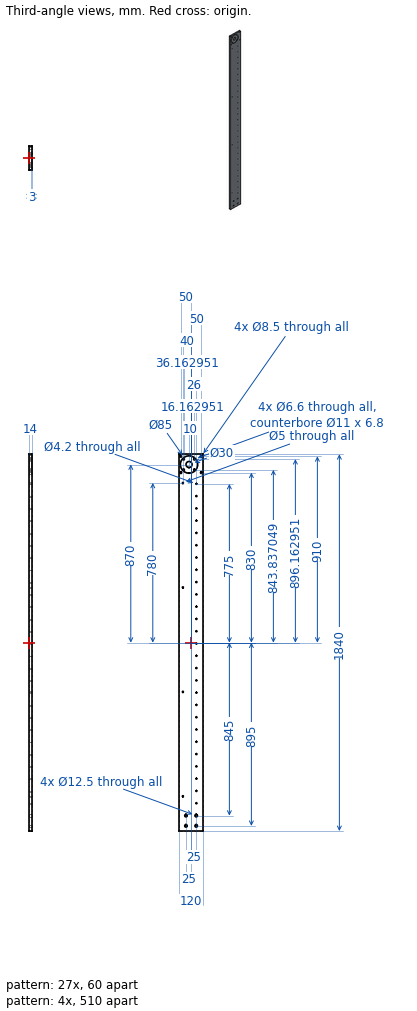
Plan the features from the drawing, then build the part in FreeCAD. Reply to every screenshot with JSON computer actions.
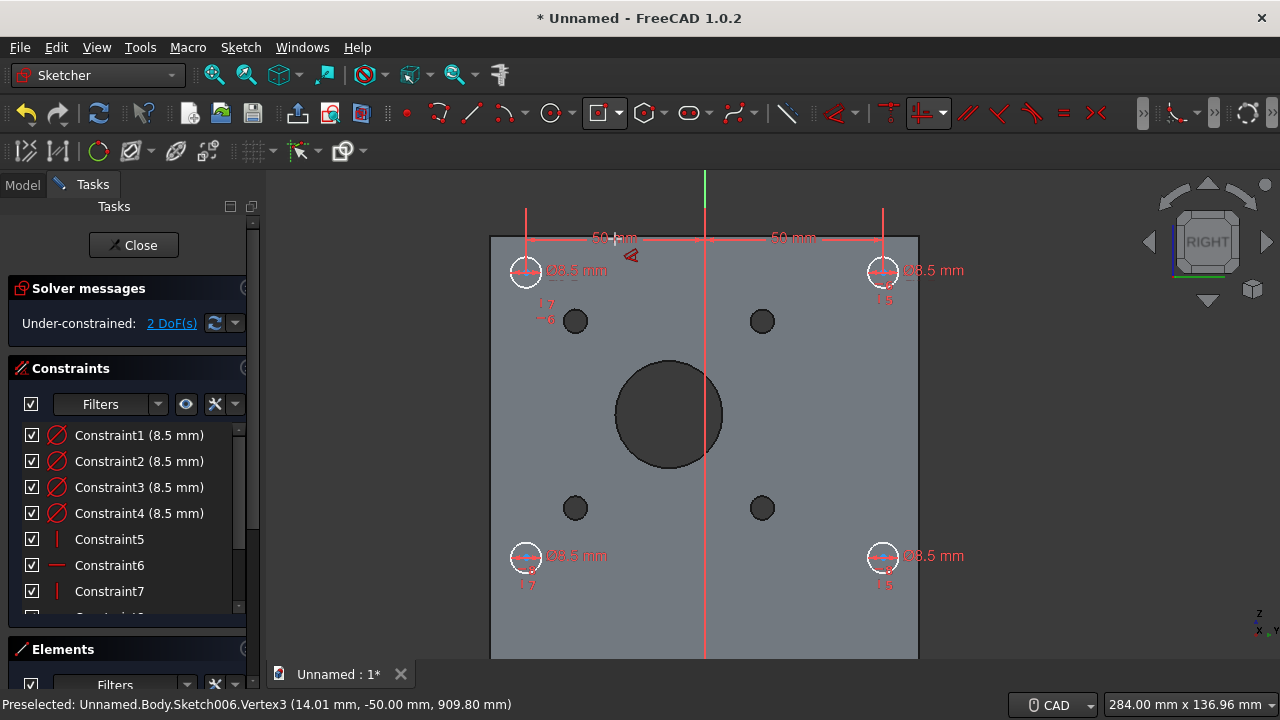
{"action": "left_click", "coordinate": [883, 273]}
{"action": "left_click", "coordinate": [917, 452]}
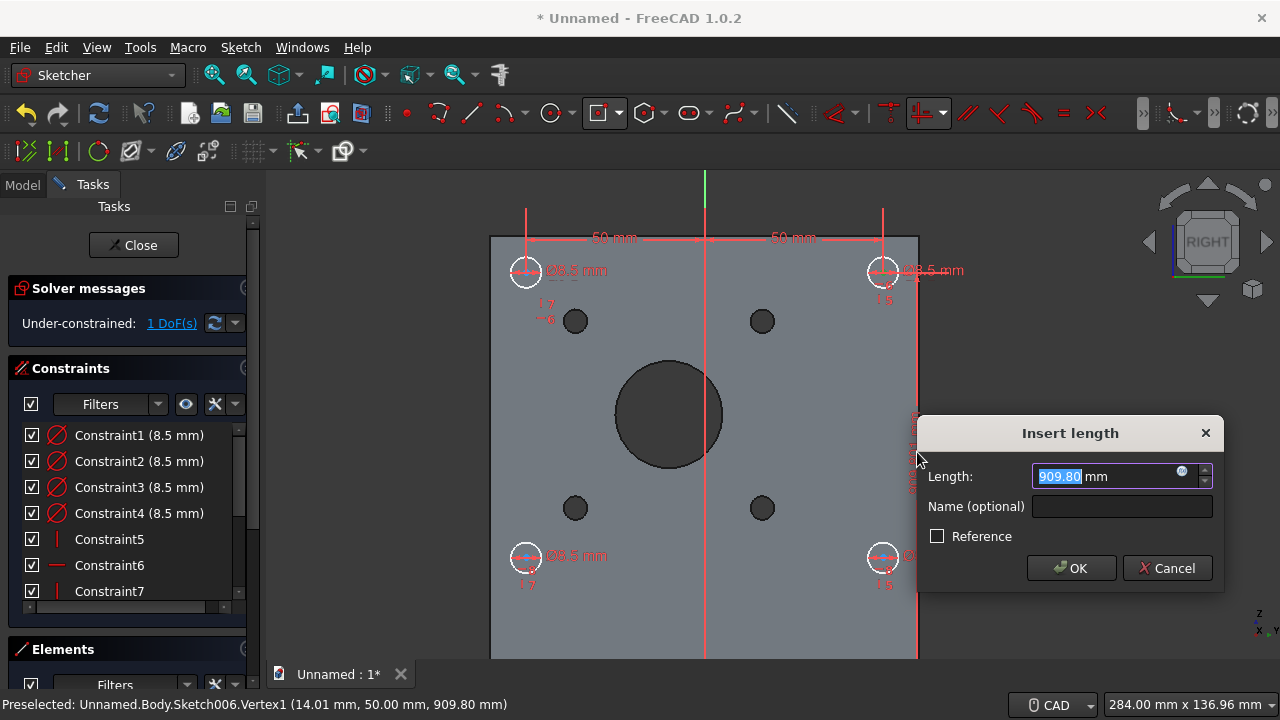
{"action": "type", "text": "910"}
{"action": "key", "text": "Return"}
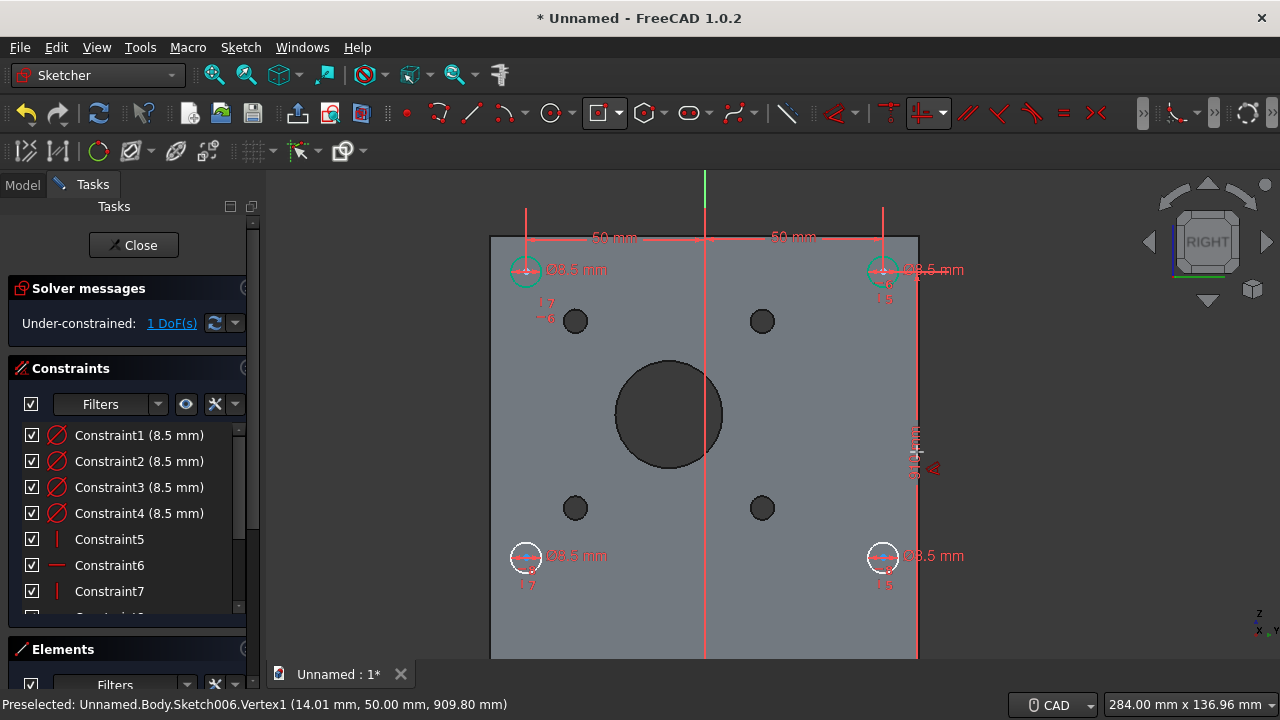
{"action": "left_click", "coordinate": [883, 558]}
{"action": "left_click", "coordinate": [917, 594]}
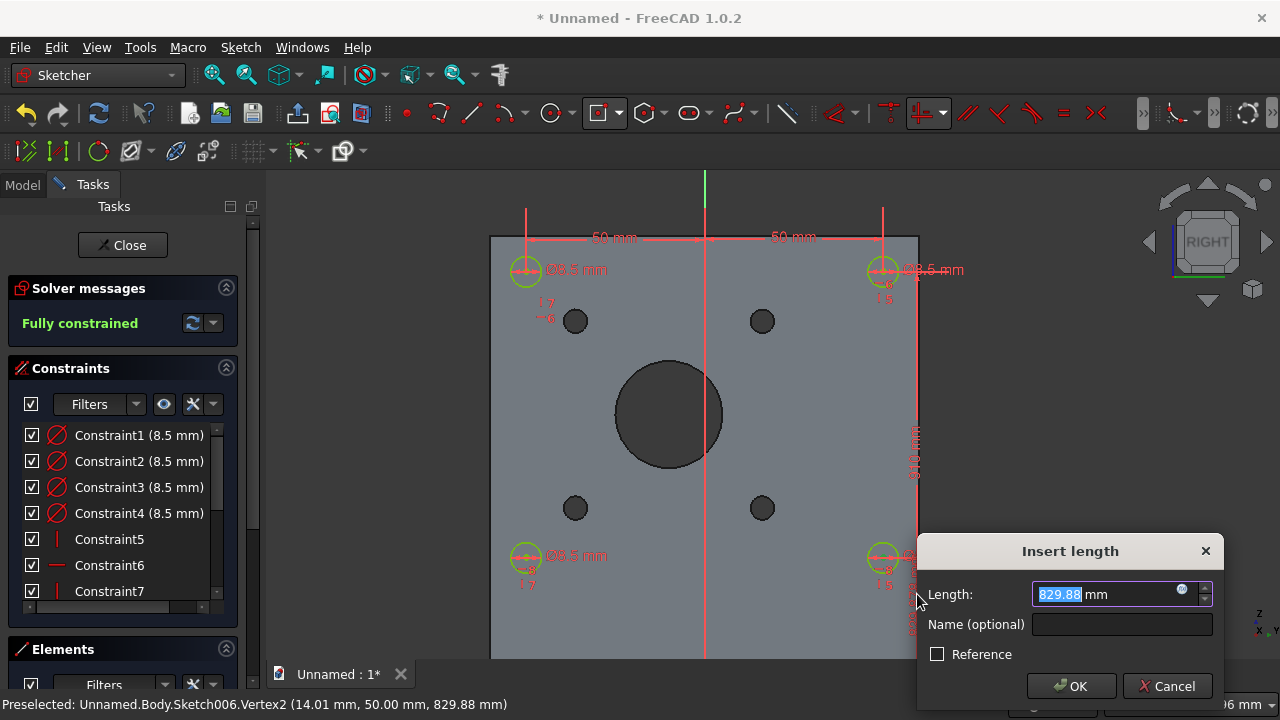
{"action": "type", "text": "830"}
{"action": "key", "text": "Return"}
{"action": "key", "text": "Escape"}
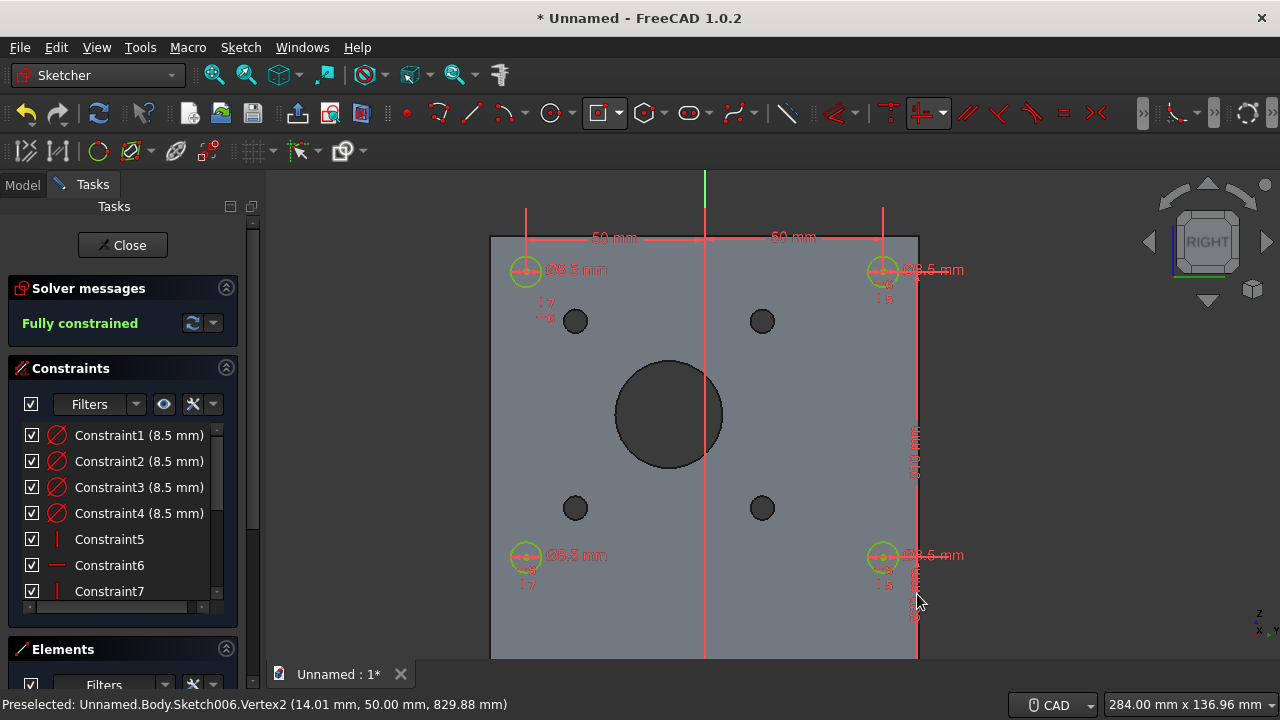
{"action": "left_click", "coordinate": [123, 245]}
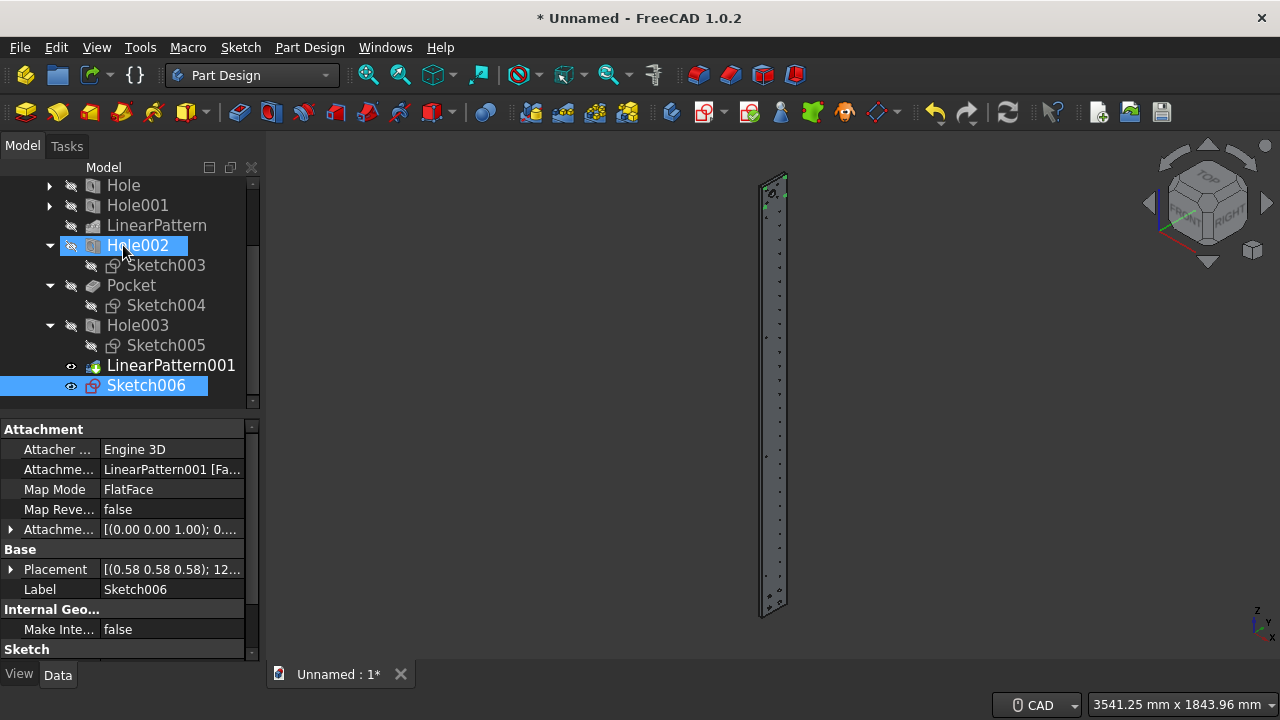
{"action": "left_click", "coordinate": [272, 112]}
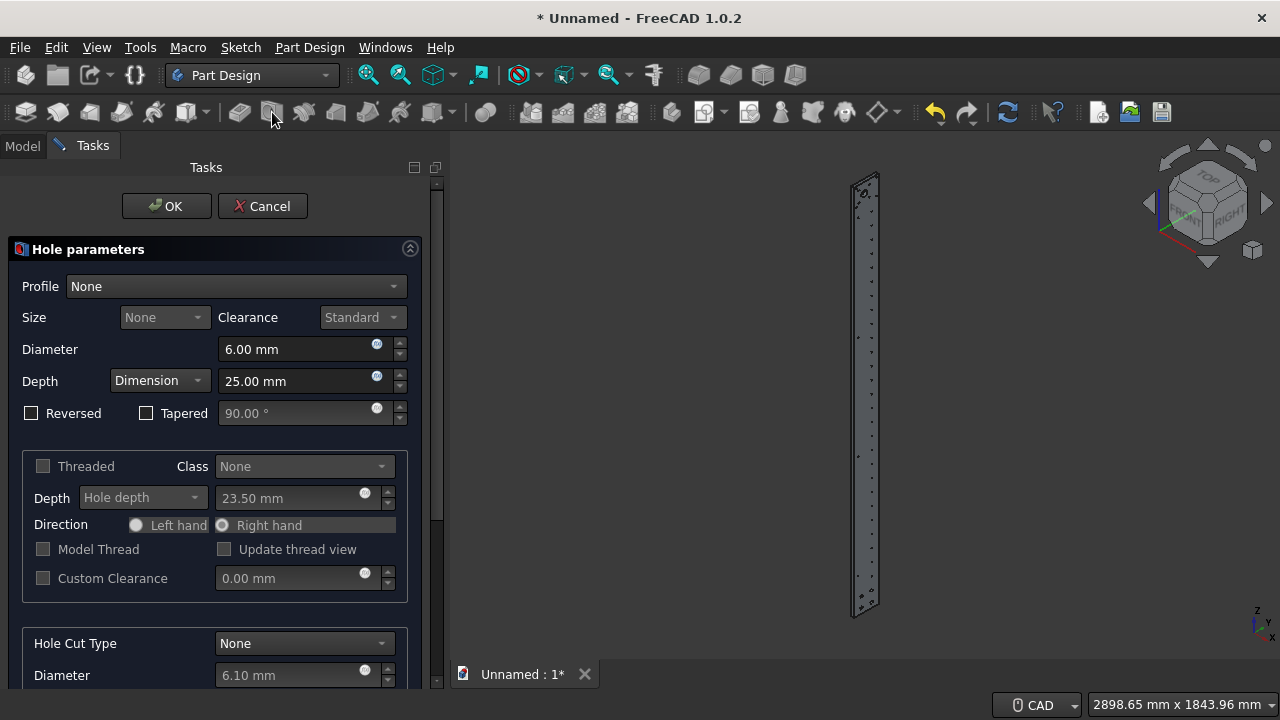
{"action": "triple_click", "coordinate": [305, 349]}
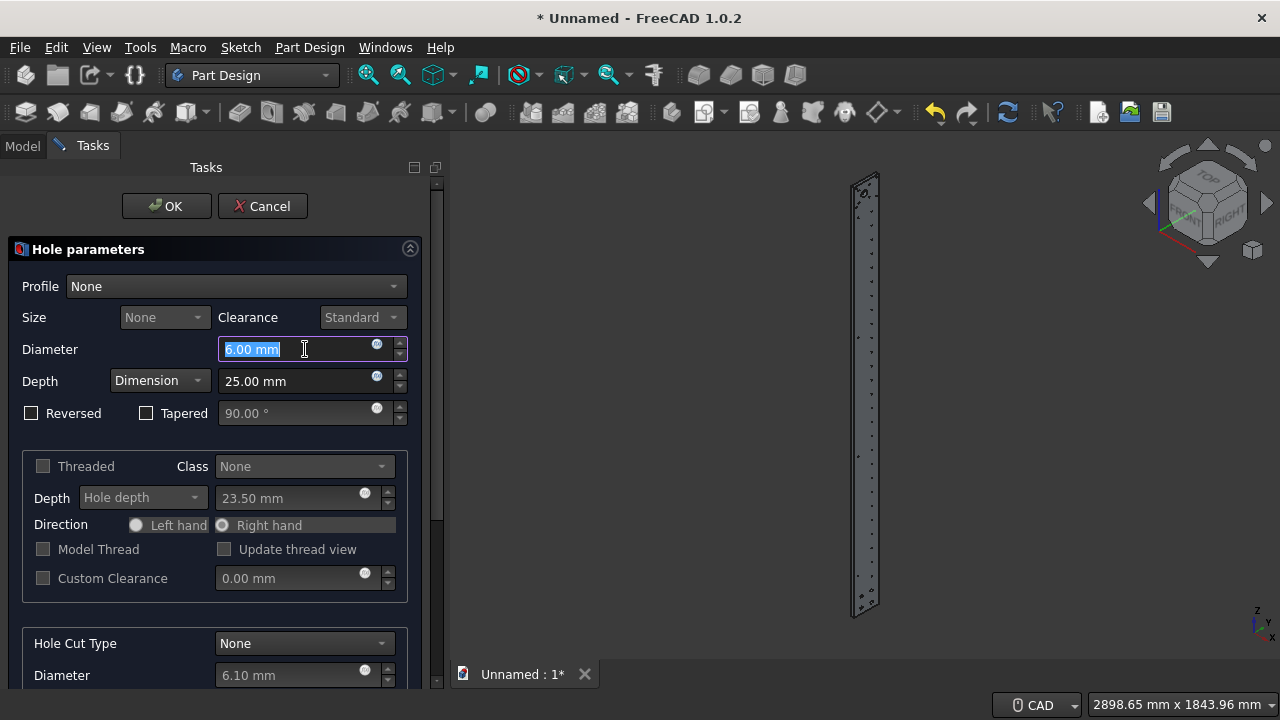
{"action": "type", "text": "8.5"}
{"action": "key", "text": "Tab"}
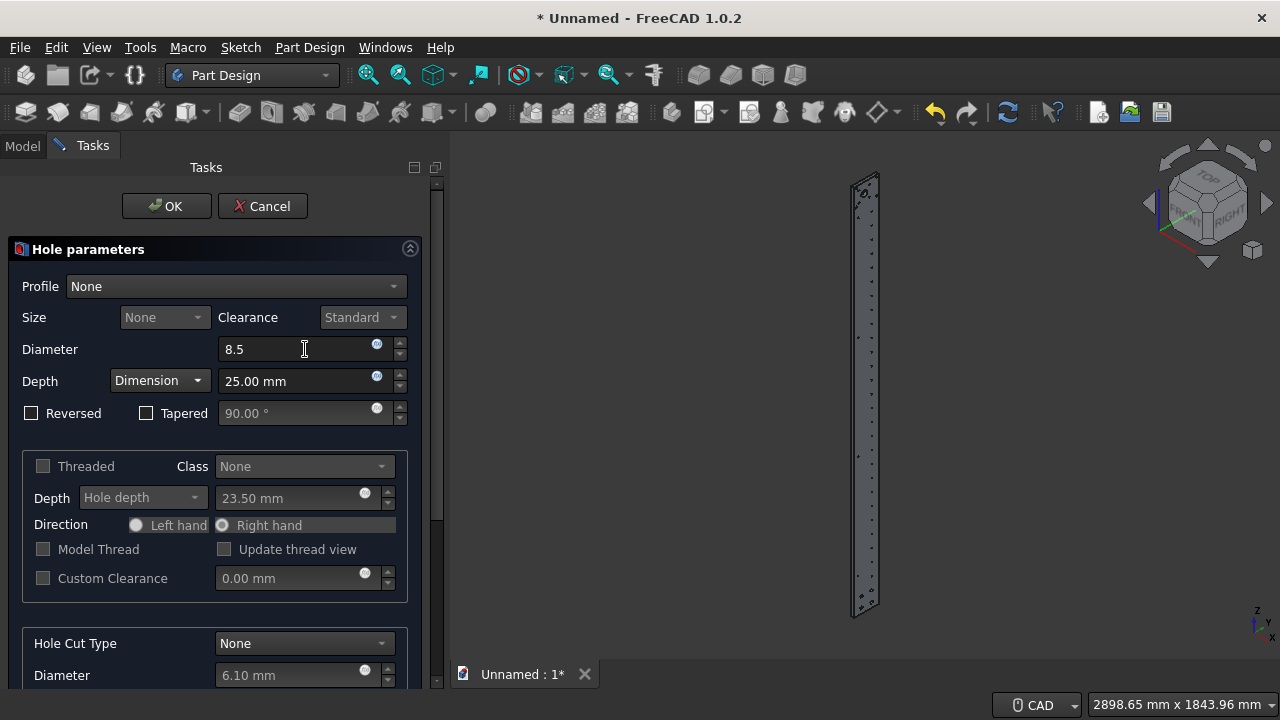
{"action": "left_click", "coordinate": [161, 380]}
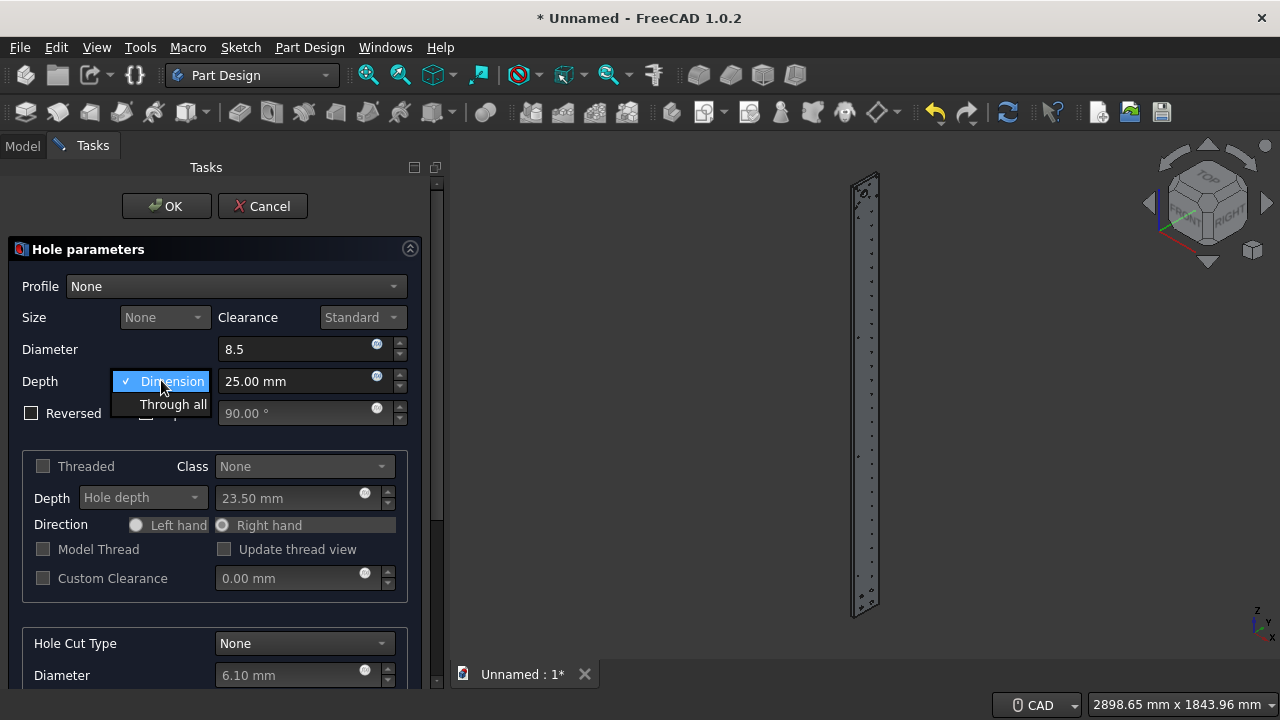
{"action": "left_click", "coordinate": [160, 404]}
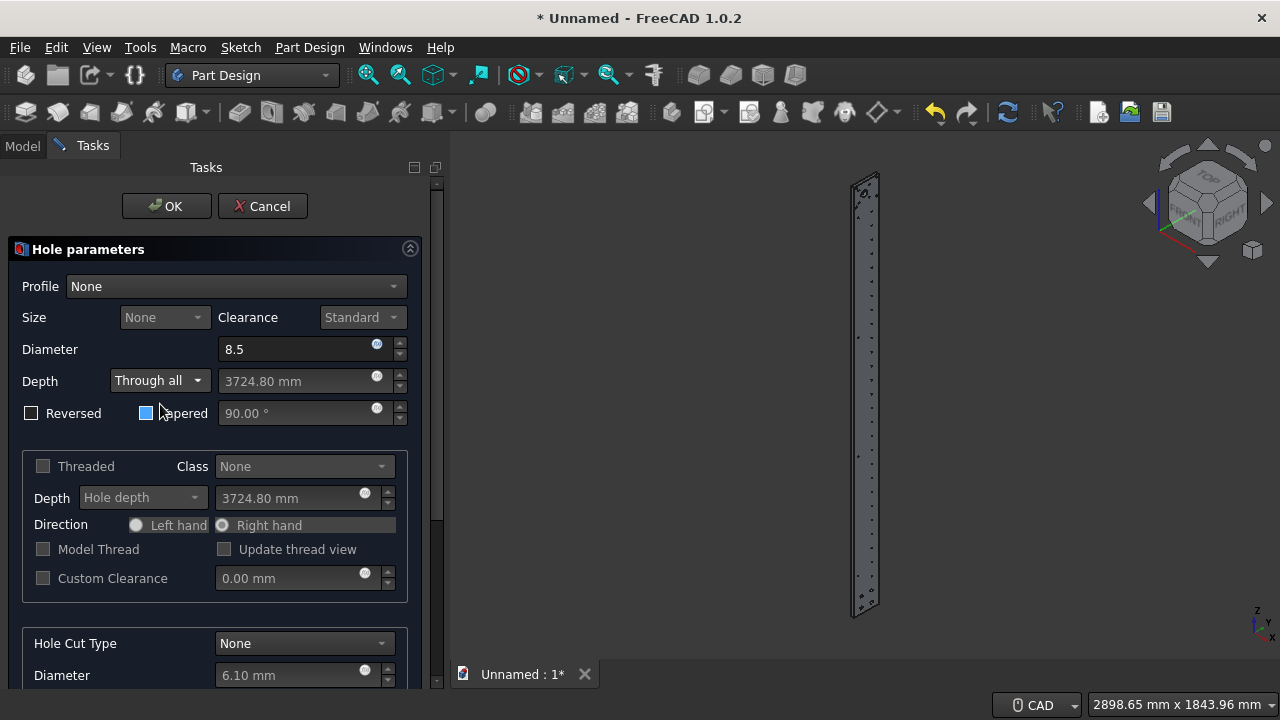
{"action": "left_click", "coordinate": [167, 206]}